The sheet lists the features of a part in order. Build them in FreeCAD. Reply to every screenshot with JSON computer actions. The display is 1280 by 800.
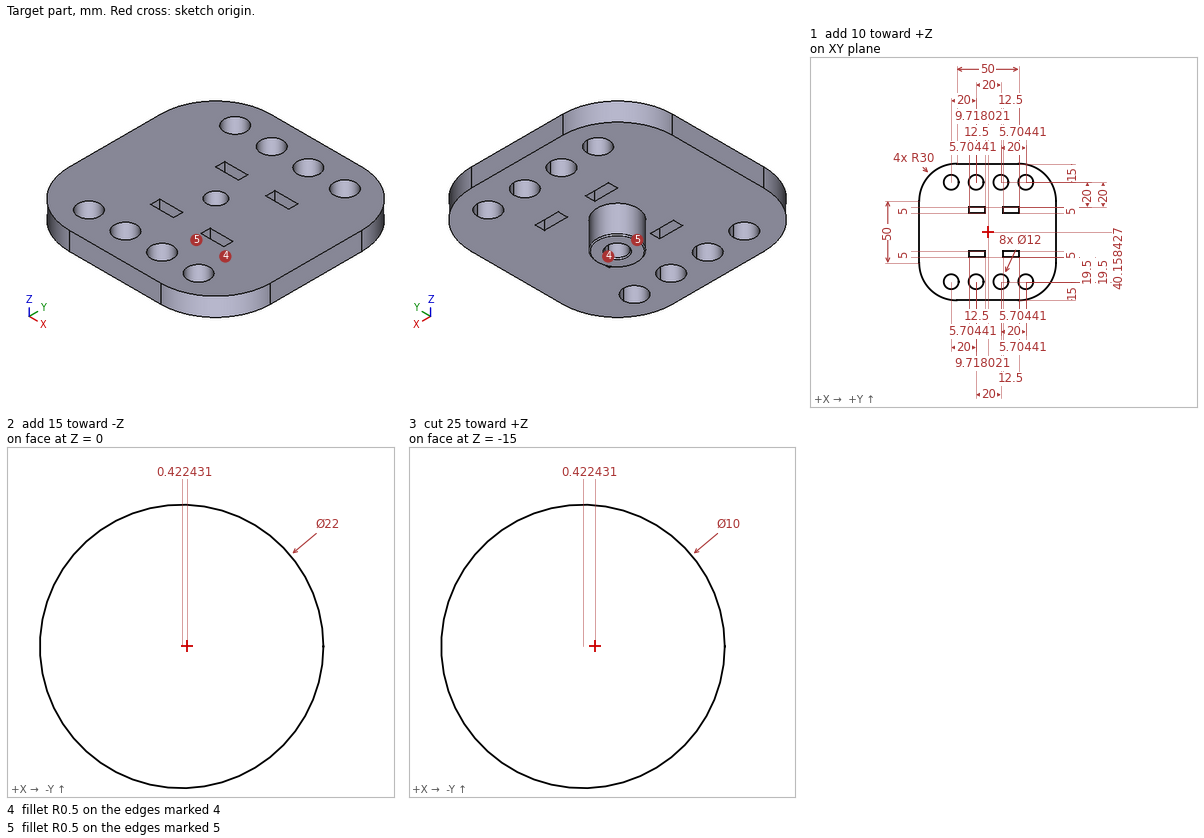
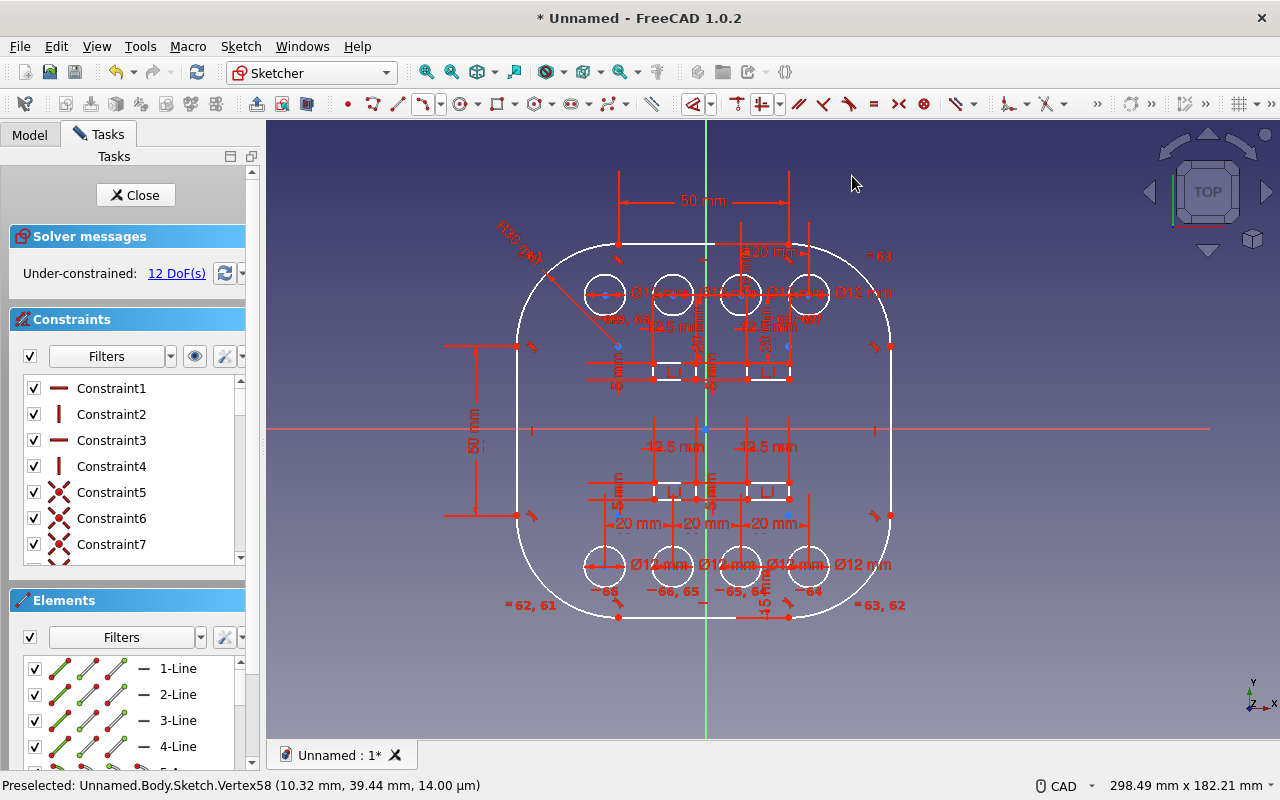
{"action": "left_click", "coordinate": [741, 295]}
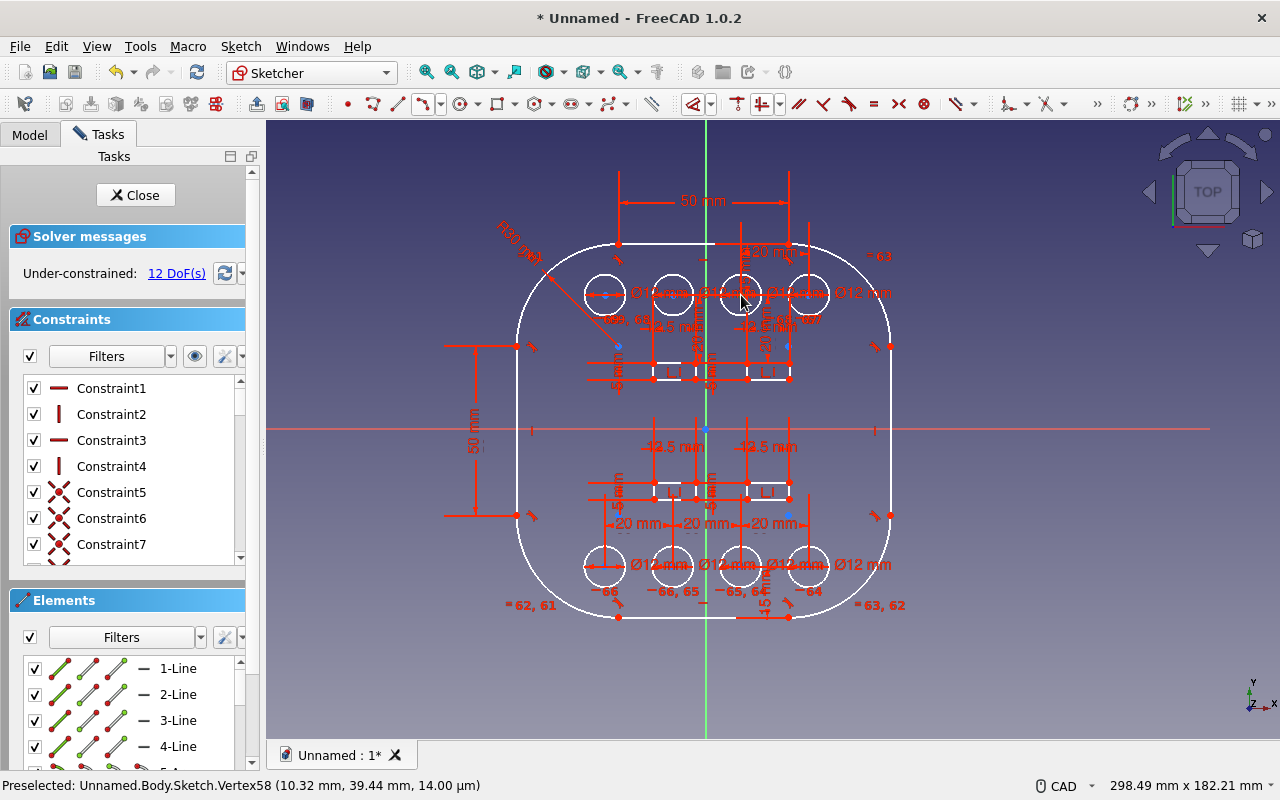
{"action": "left_click", "coordinate": [673, 295]}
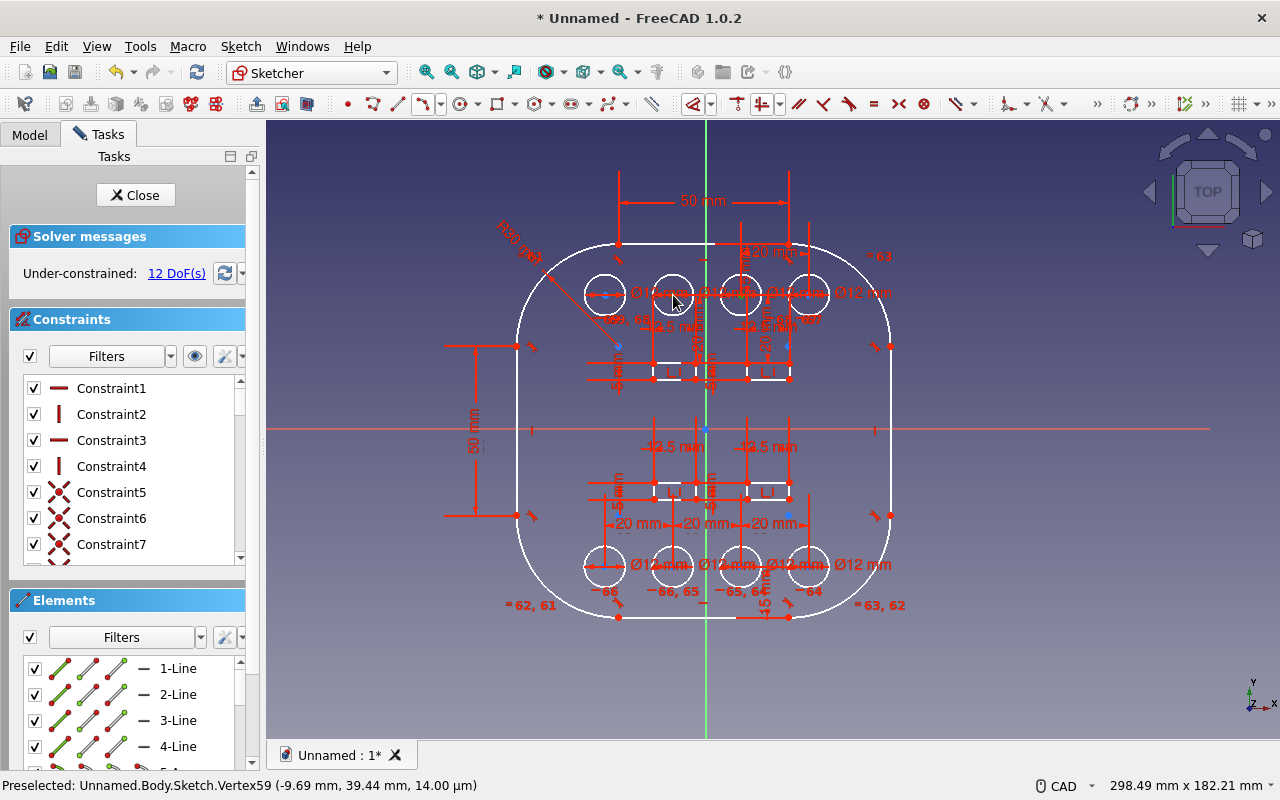
{"action": "key", "text": "l"}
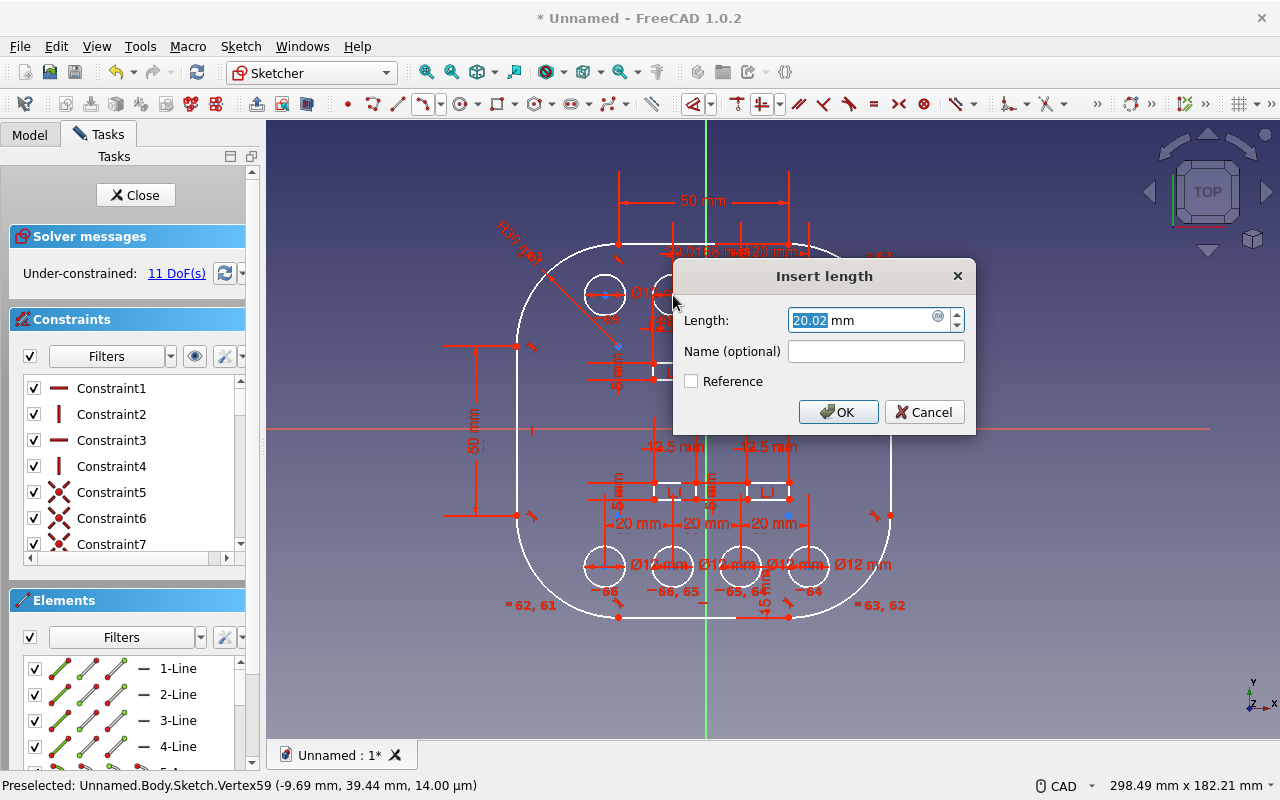
{"action": "type", "text": "20"}
{"action": "key", "text": "Return"}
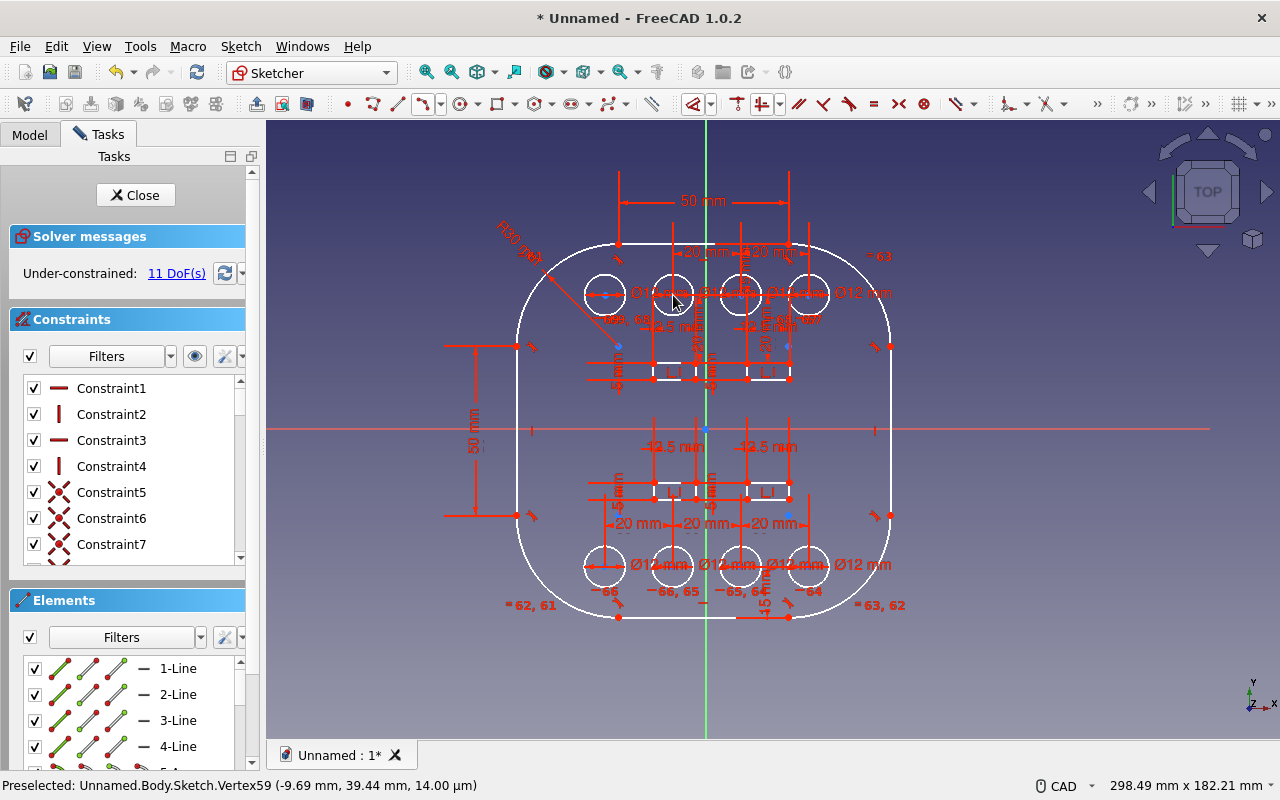
{"action": "left_click", "coordinate": [673, 295]}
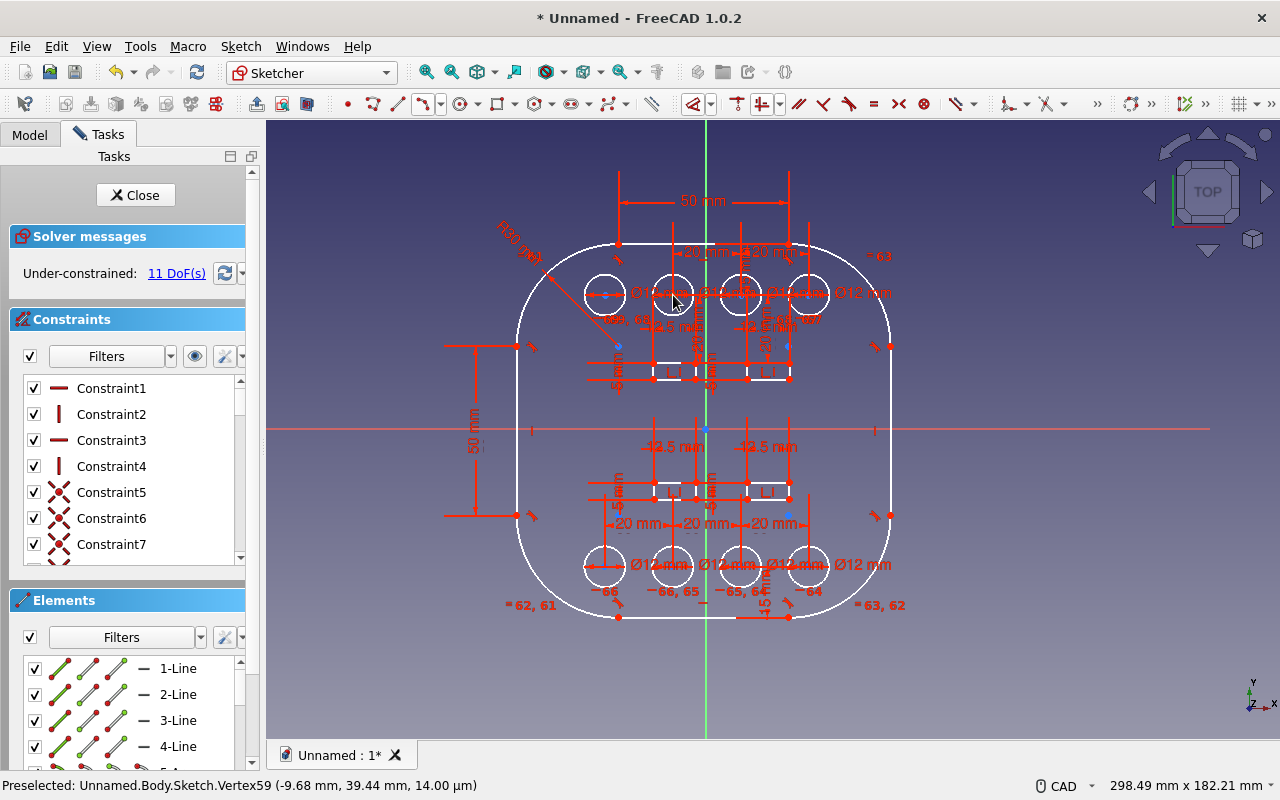
{"action": "left_click", "coordinate": [605, 295]}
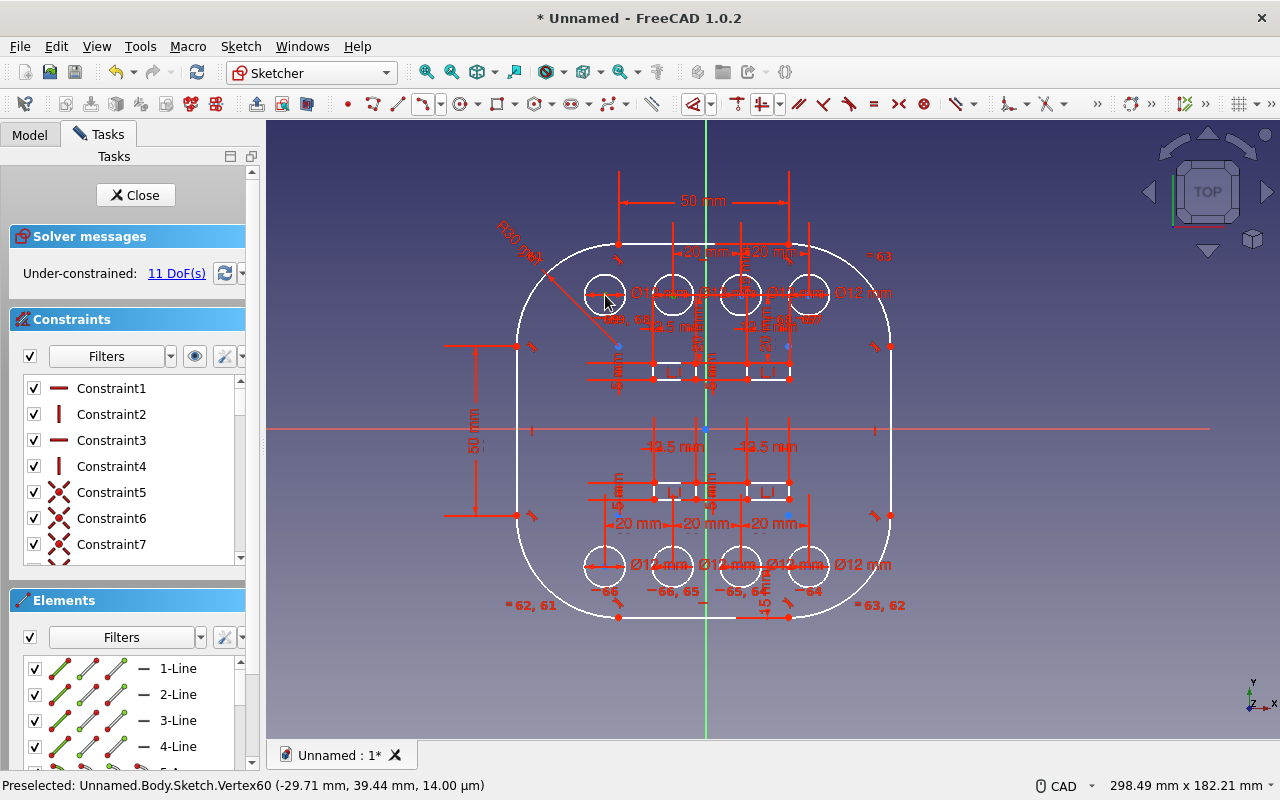
{"action": "key", "text": "l"}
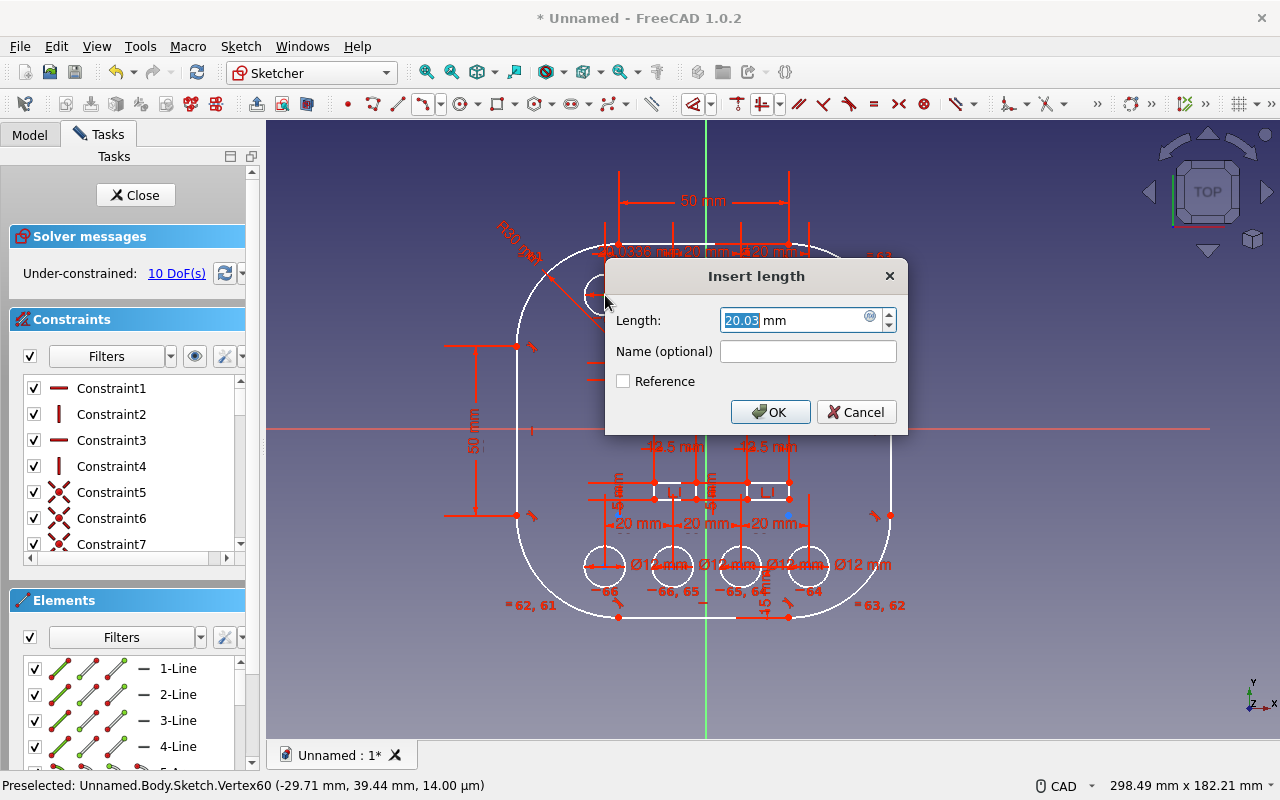
{"action": "type", "text": "20"}
{"action": "key", "text": "Return"}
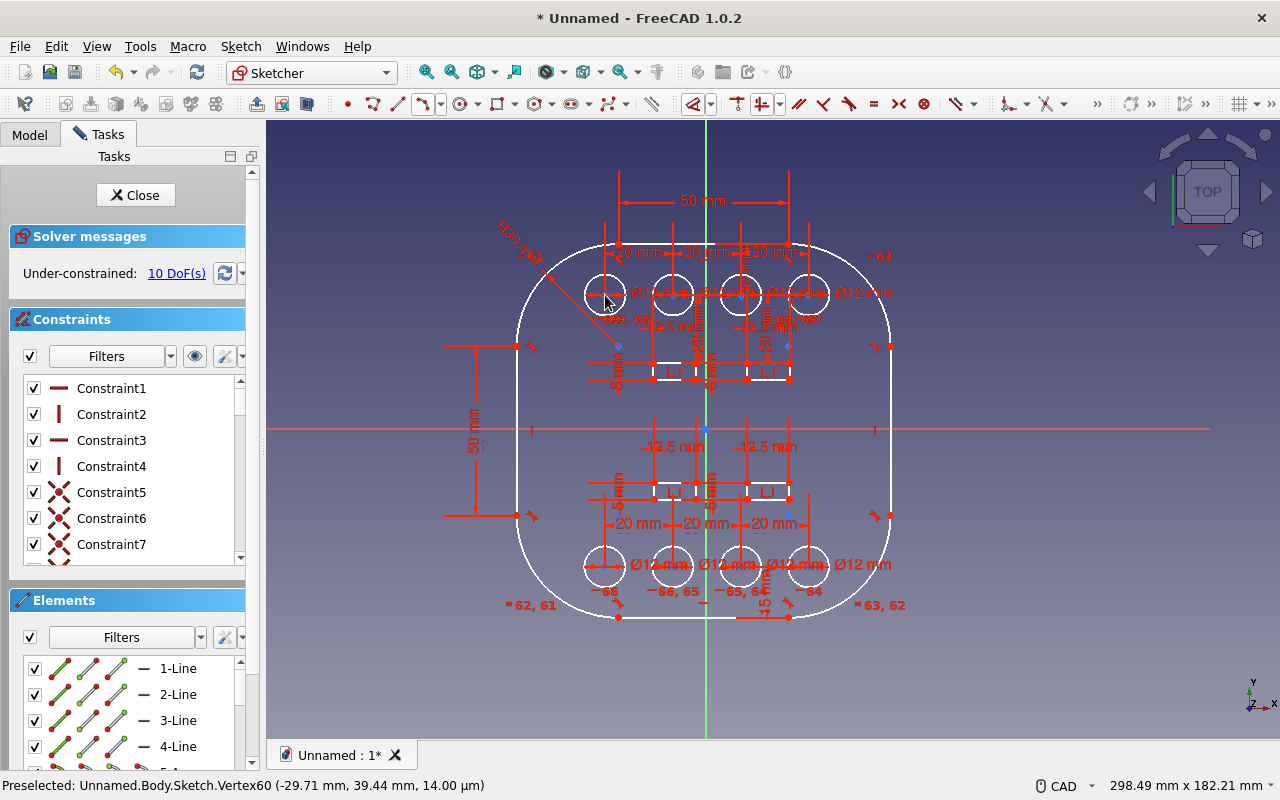
{"action": "left_click", "coordinate": [789, 500]}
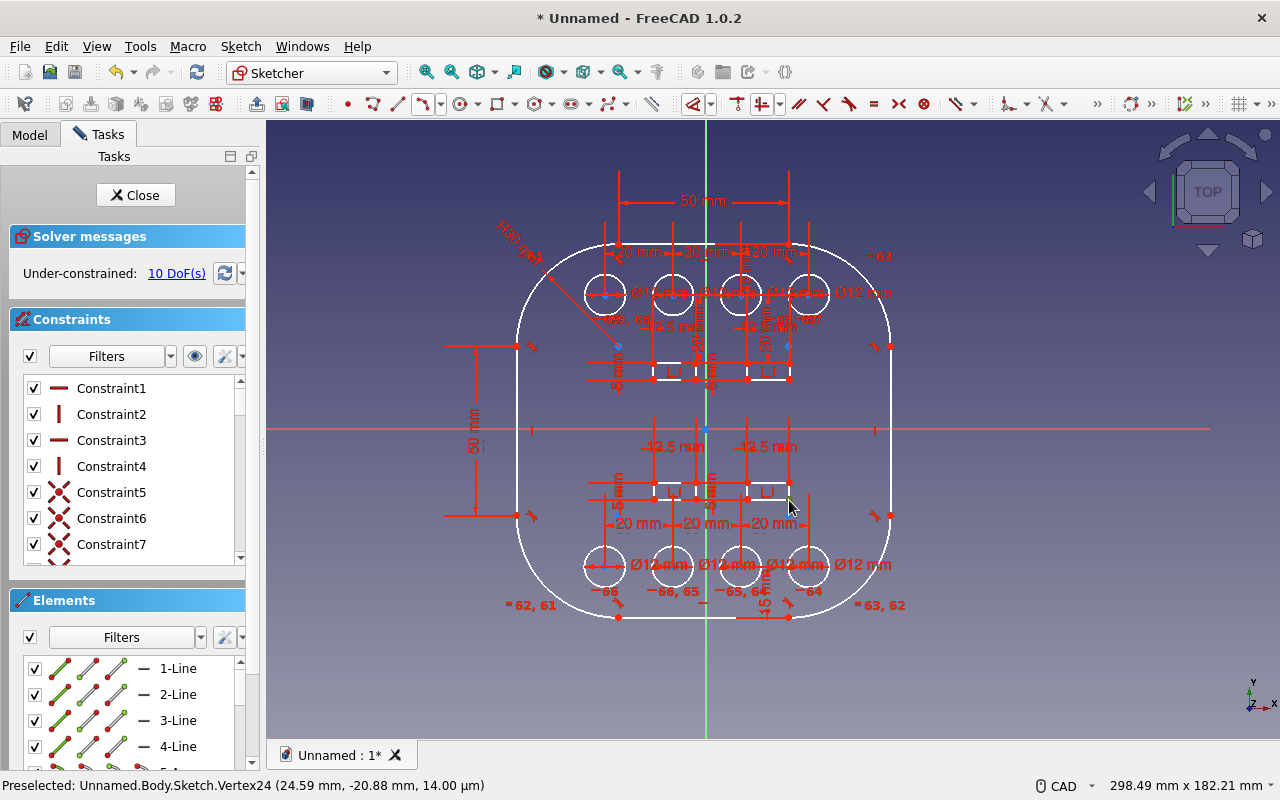
{"action": "left_click", "coordinate": [809, 567]}